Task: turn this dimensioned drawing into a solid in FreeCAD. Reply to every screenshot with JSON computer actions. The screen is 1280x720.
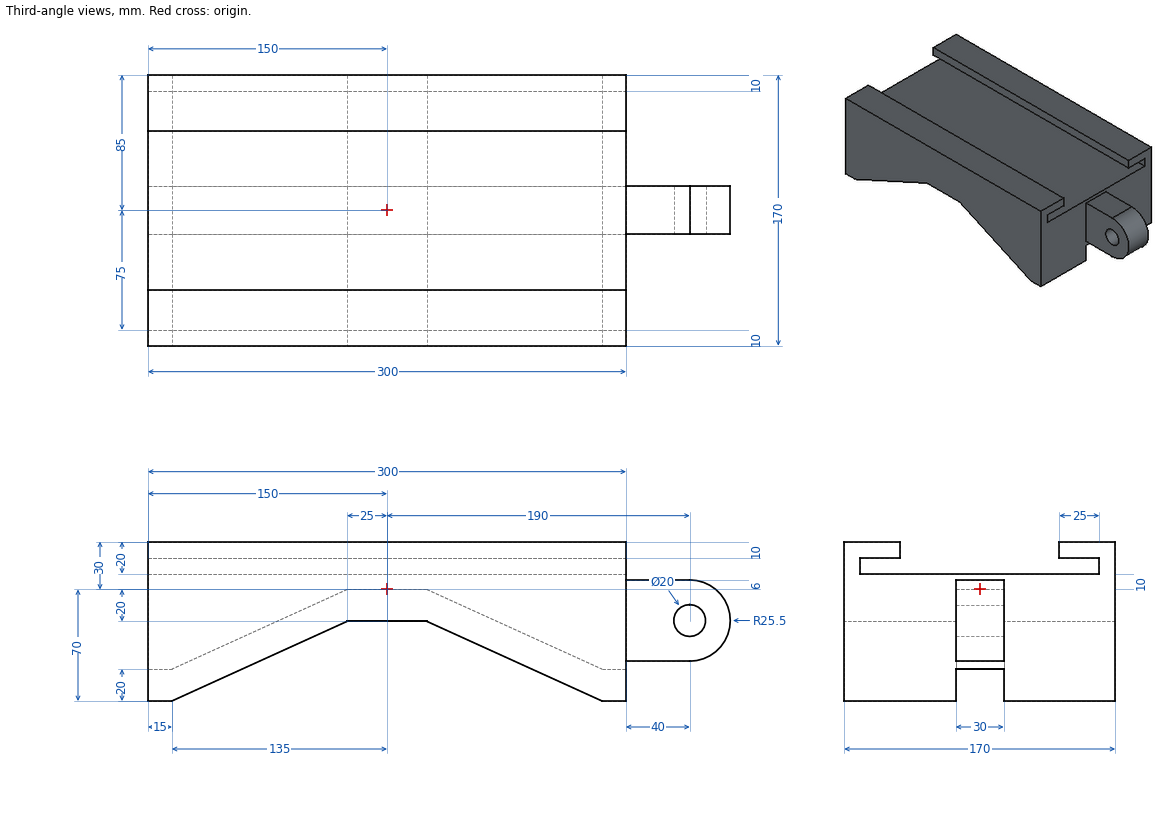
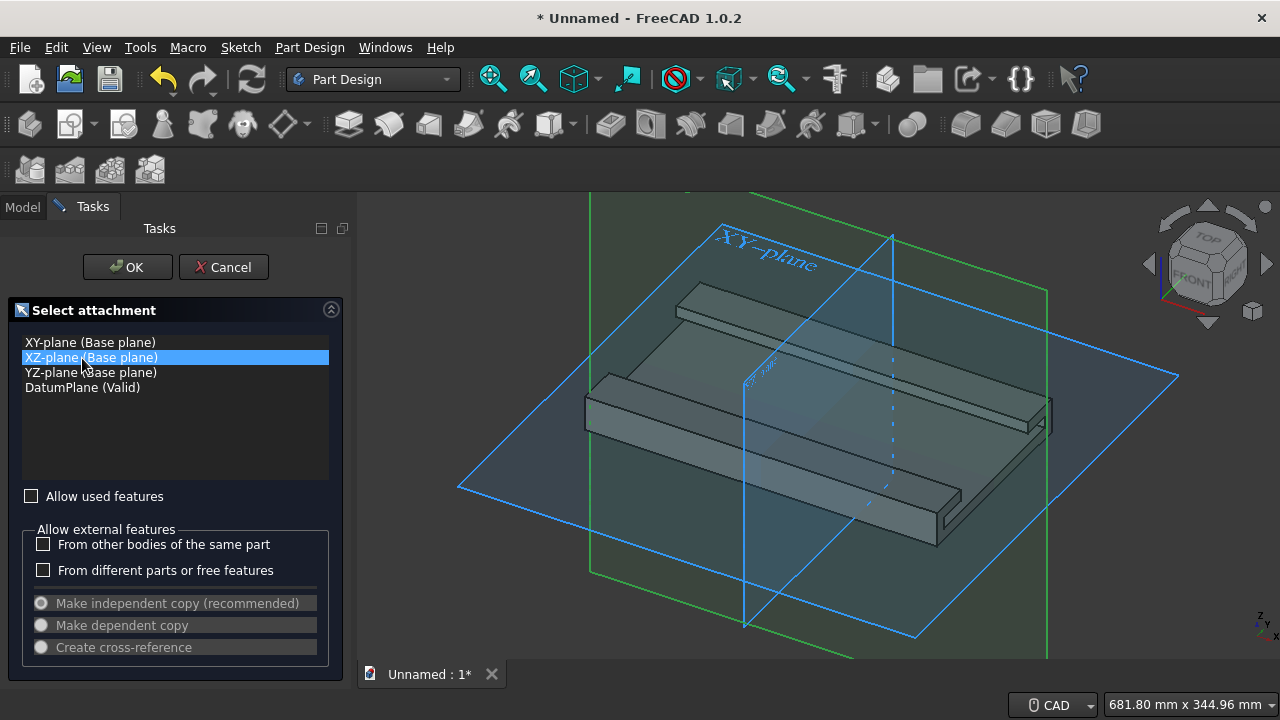
{"action": "left_click", "coordinate": [128, 267]}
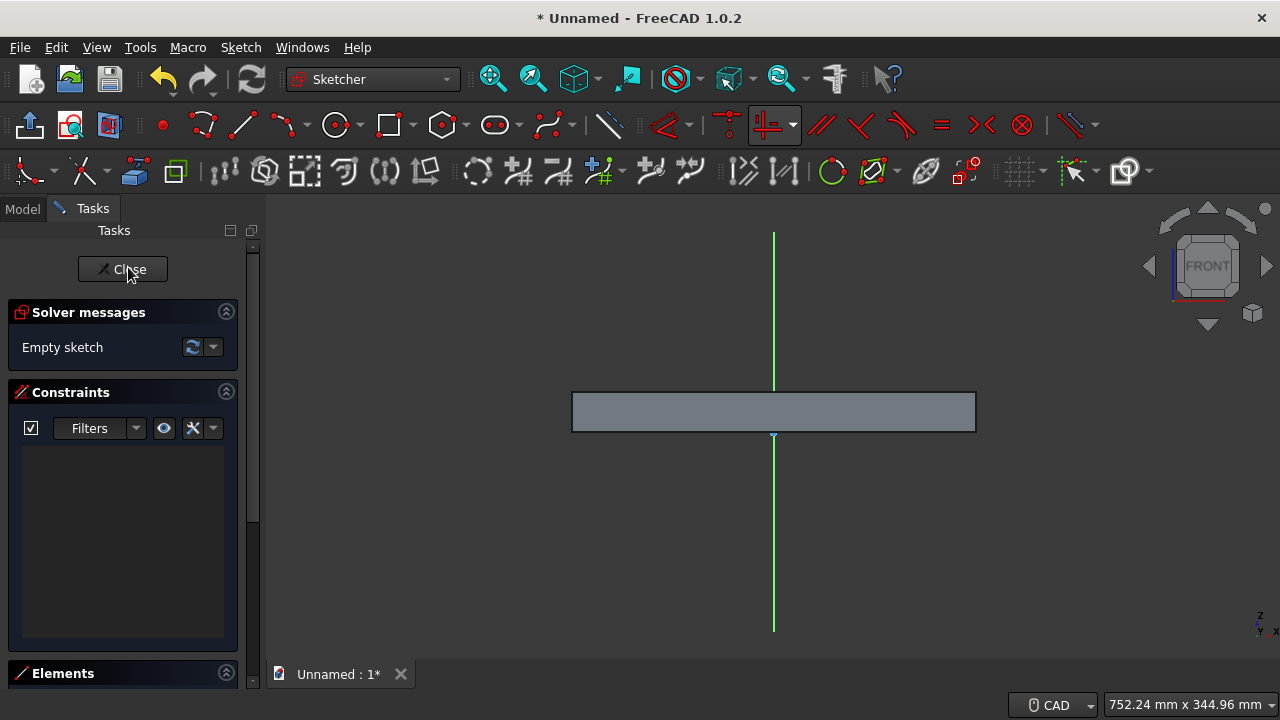
{"action": "key", "text": "q s"}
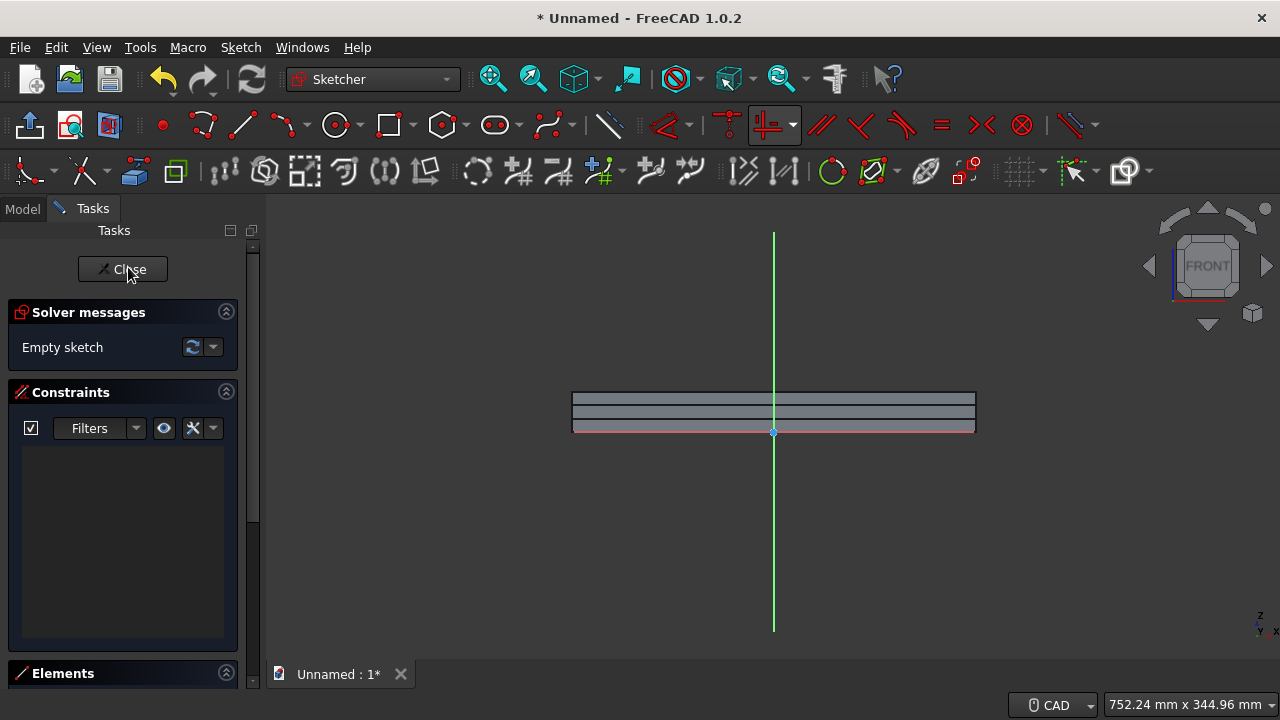
{"action": "scroll", "coordinate": [654, 510], "scroll_direction": "up", "scroll_amount": 5}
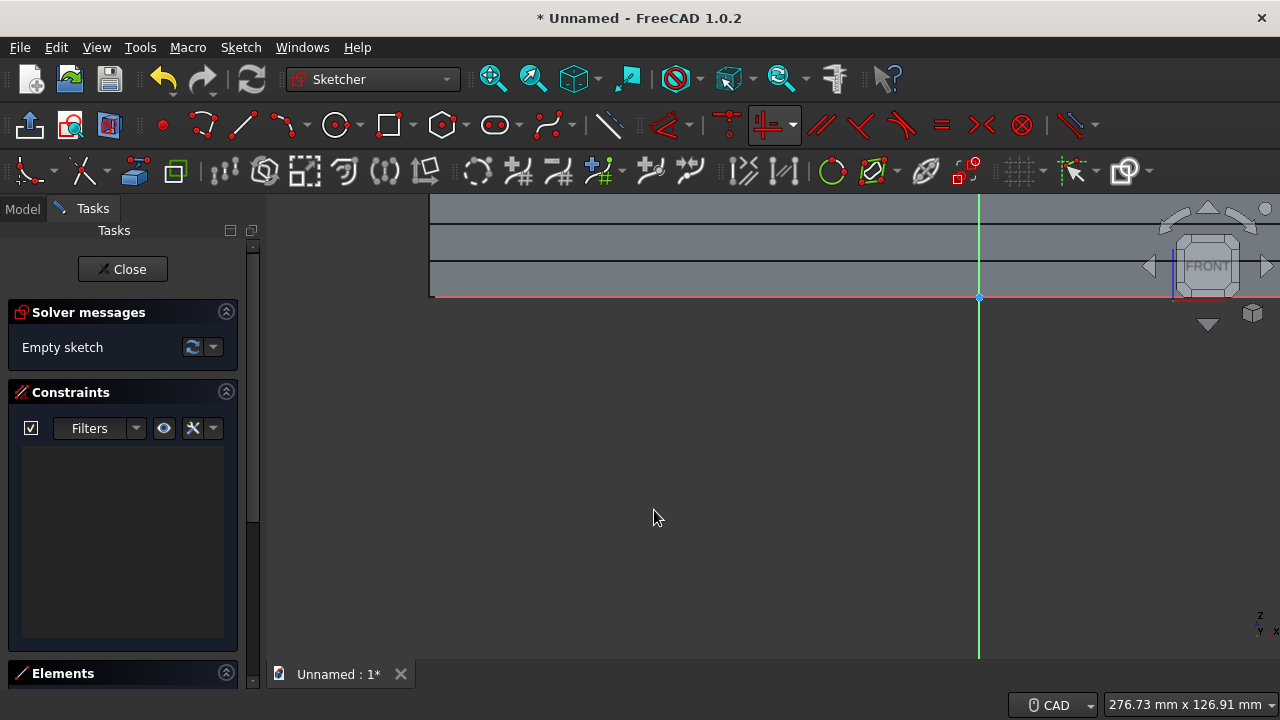
{"action": "left_click", "coordinate": [204, 126]}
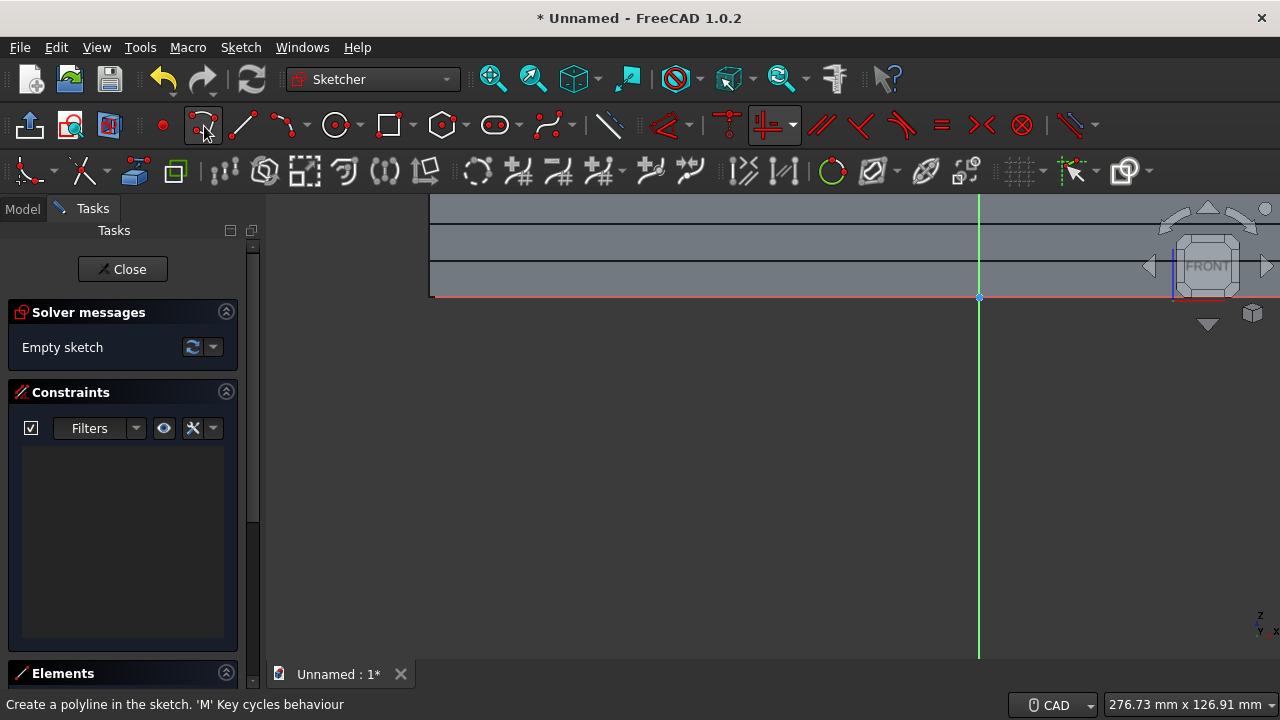
{"action": "left_click", "coordinate": [979, 297]}
{"action": "left_click", "coordinate": [970, 371]}
{"action": "left_click", "coordinate": [887, 371]}
{"action": "left_click", "coordinate": [484, 554]}
{"action": "left_click", "coordinate": [429, 554]}
{"action": "left_click", "coordinate": [429, 306]}
{"action": "left_click", "coordinate": [979, 297]}
{"action": "key", "text": "Escape"}
{"action": "key", "text": "Escape"}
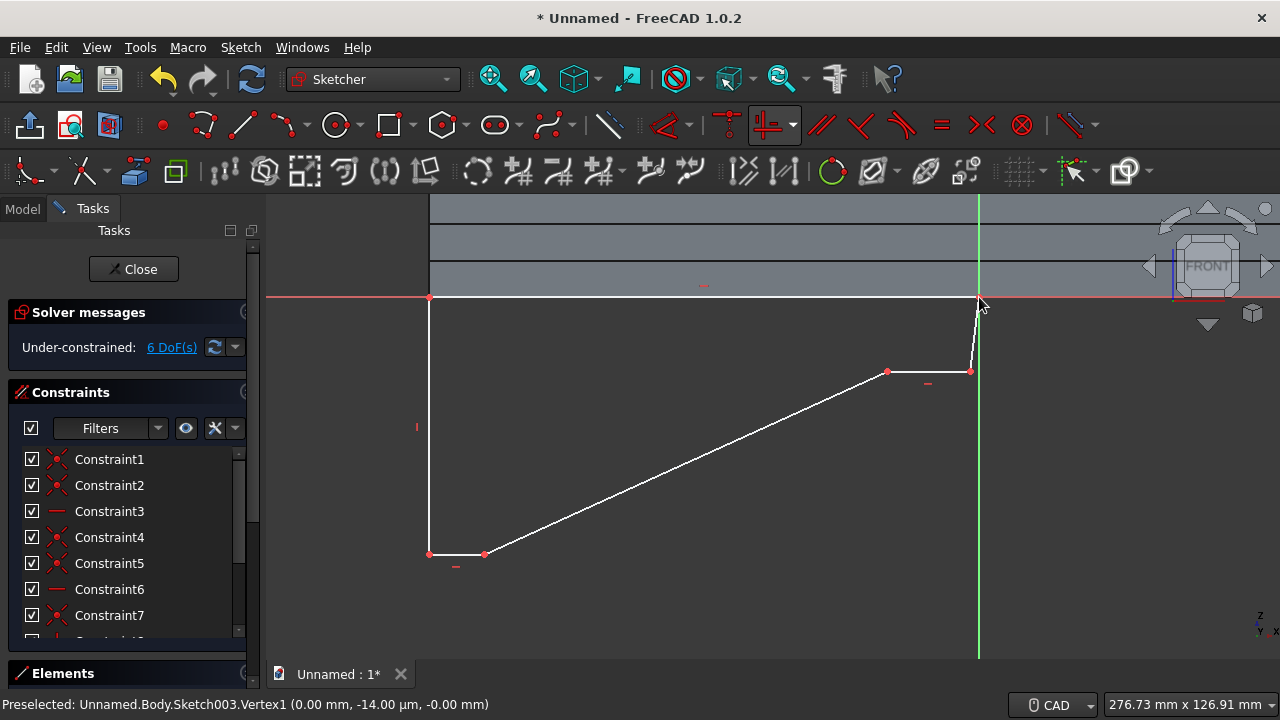
{"action": "left_click", "coordinate": [976, 320]}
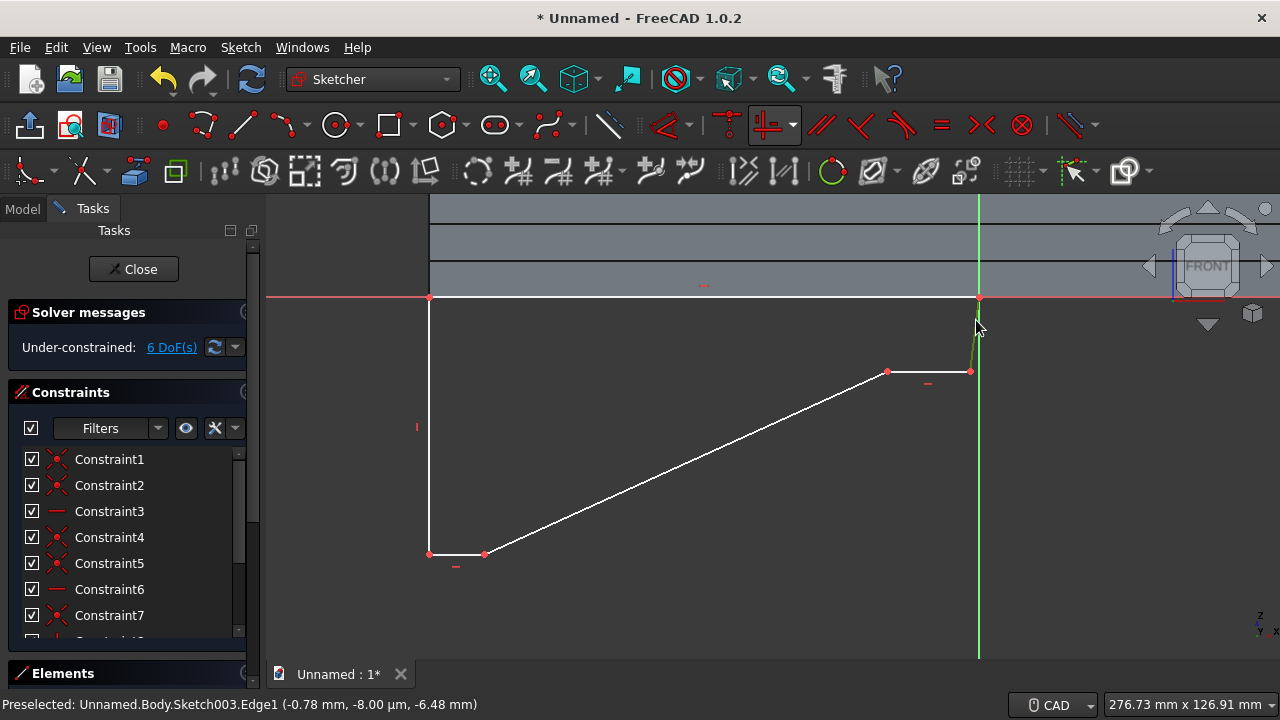
{"action": "key", "text": "v"}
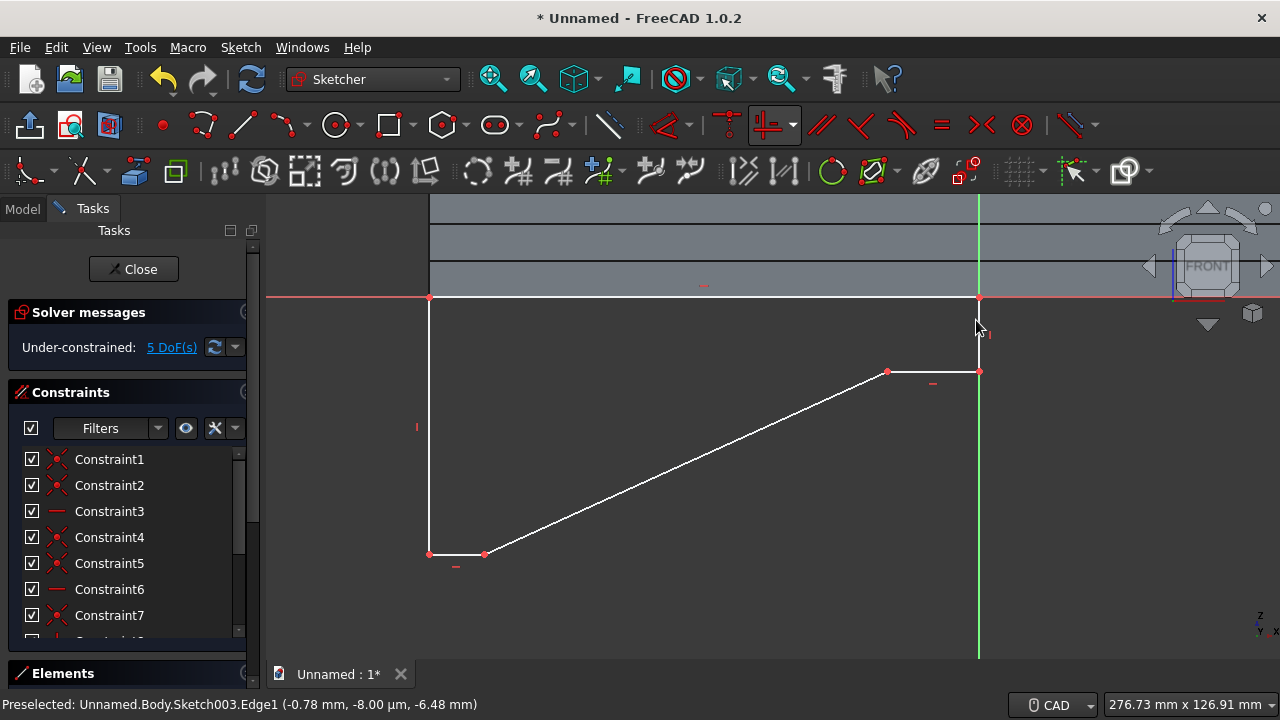
{"action": "key", "text": "d"}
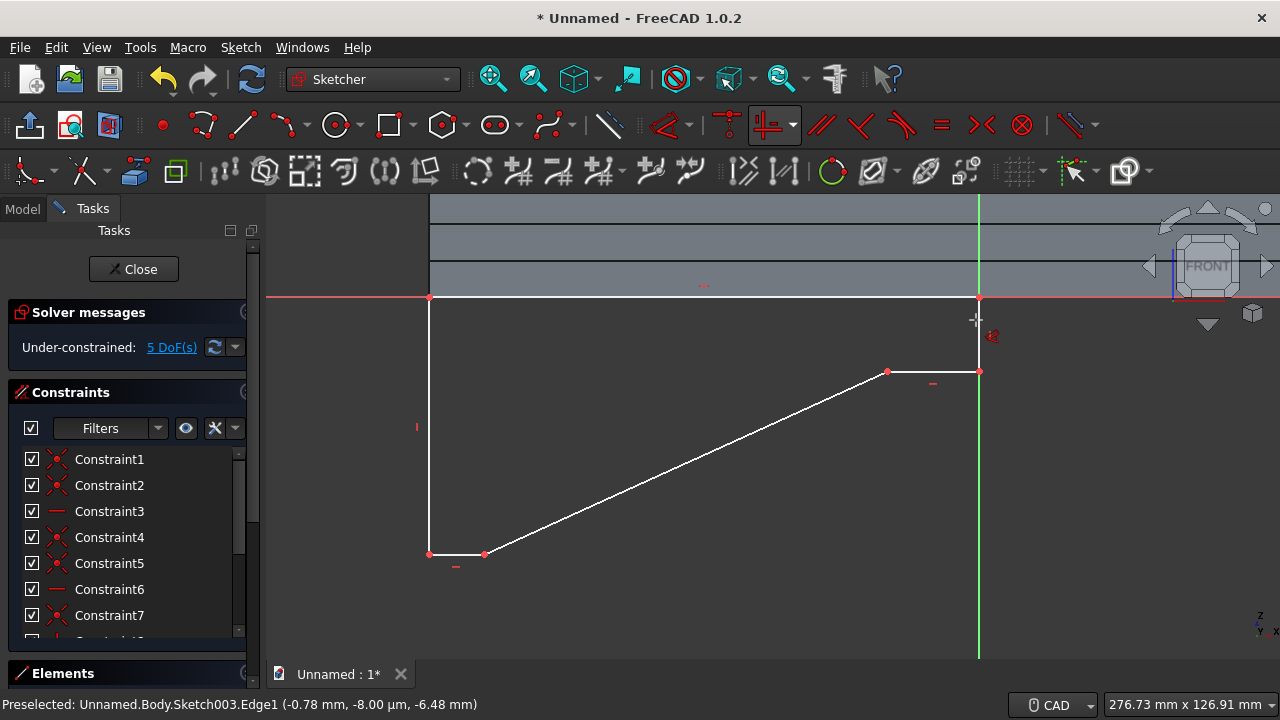
{"action": "left_click", "coordinate": [979, 320]}
{"action": "left_click", "coordinate": [1013, 335]}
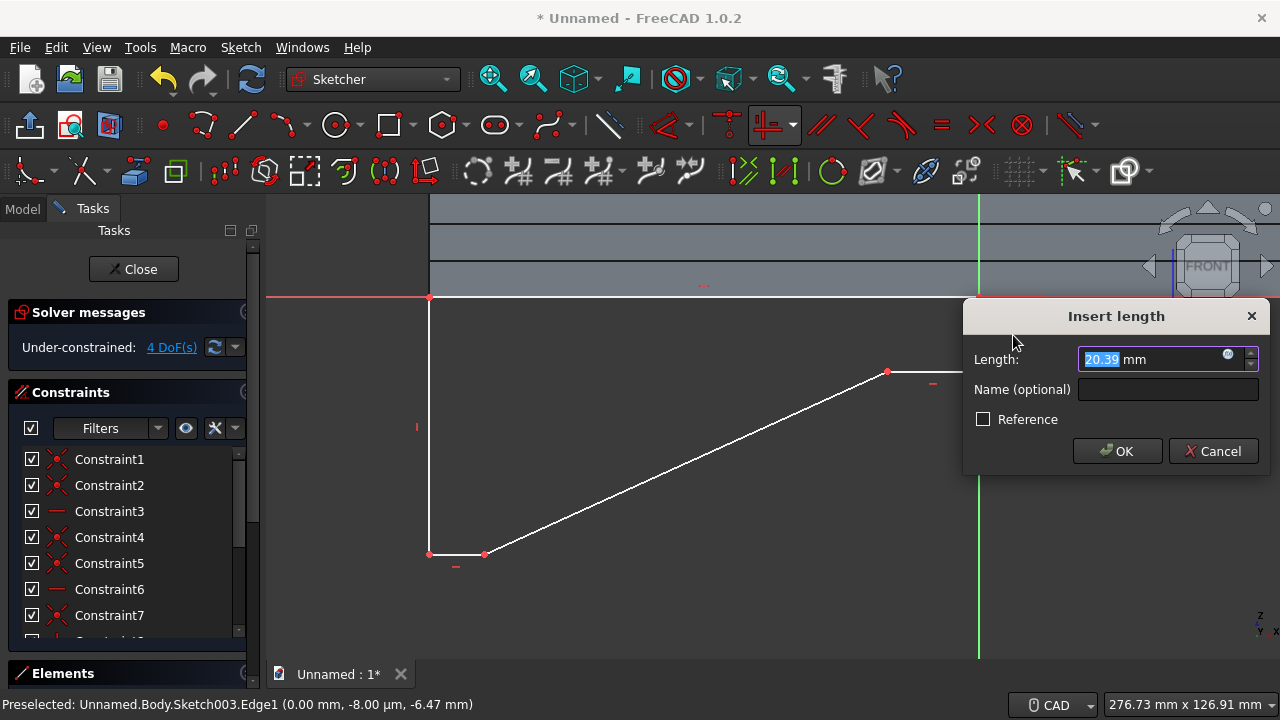
{"action": "type", "text": "20"}
{"action": "key", "text": "Return"}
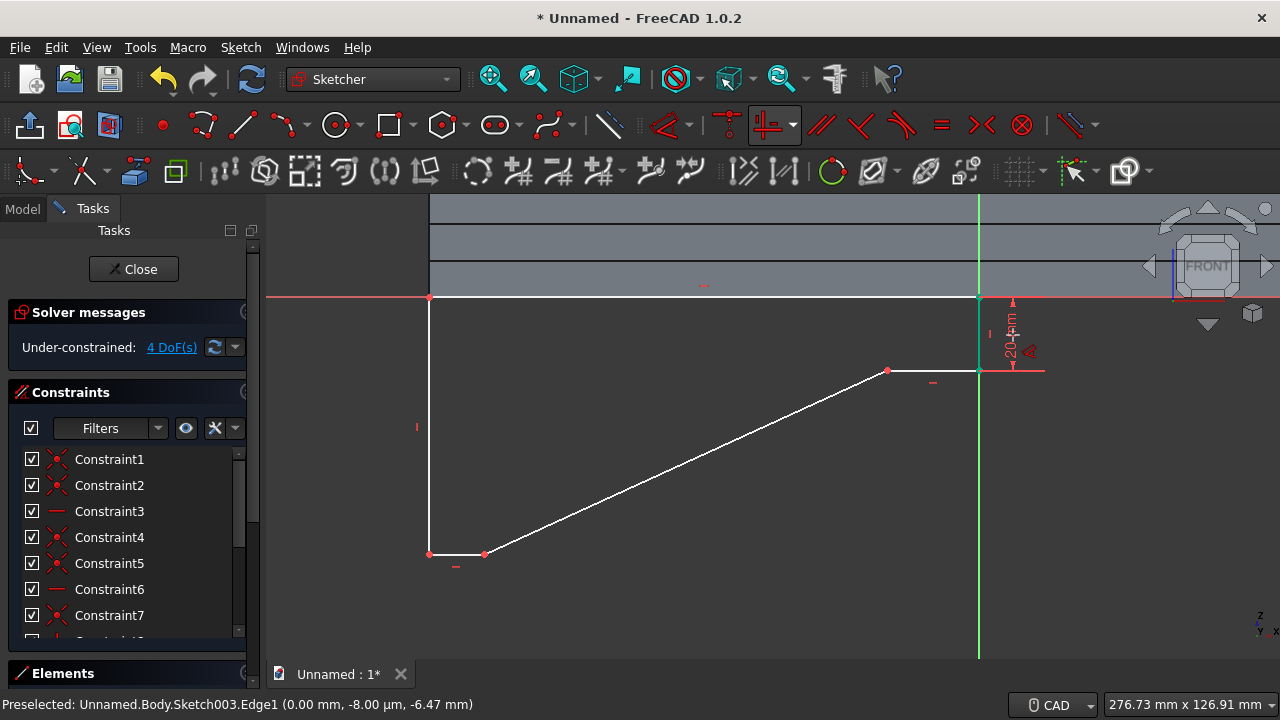
{"action": "left_click", "coordinate": [951, 371]}
{"action": "left_click", "coordinate": [933, 337]}